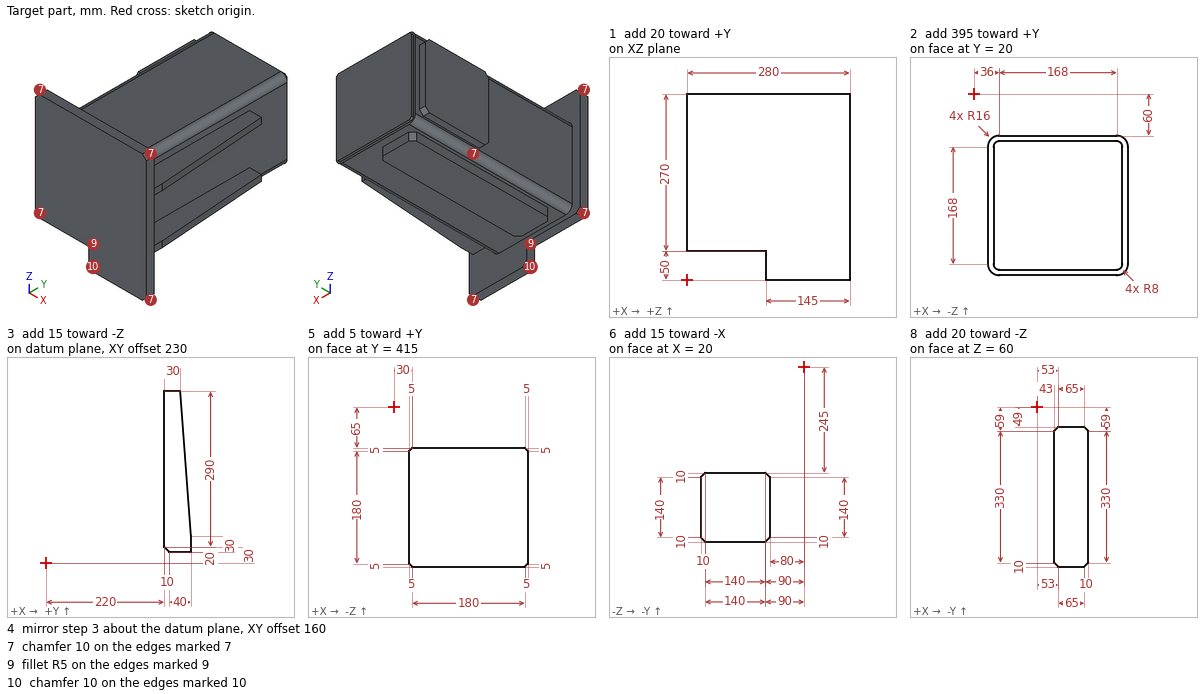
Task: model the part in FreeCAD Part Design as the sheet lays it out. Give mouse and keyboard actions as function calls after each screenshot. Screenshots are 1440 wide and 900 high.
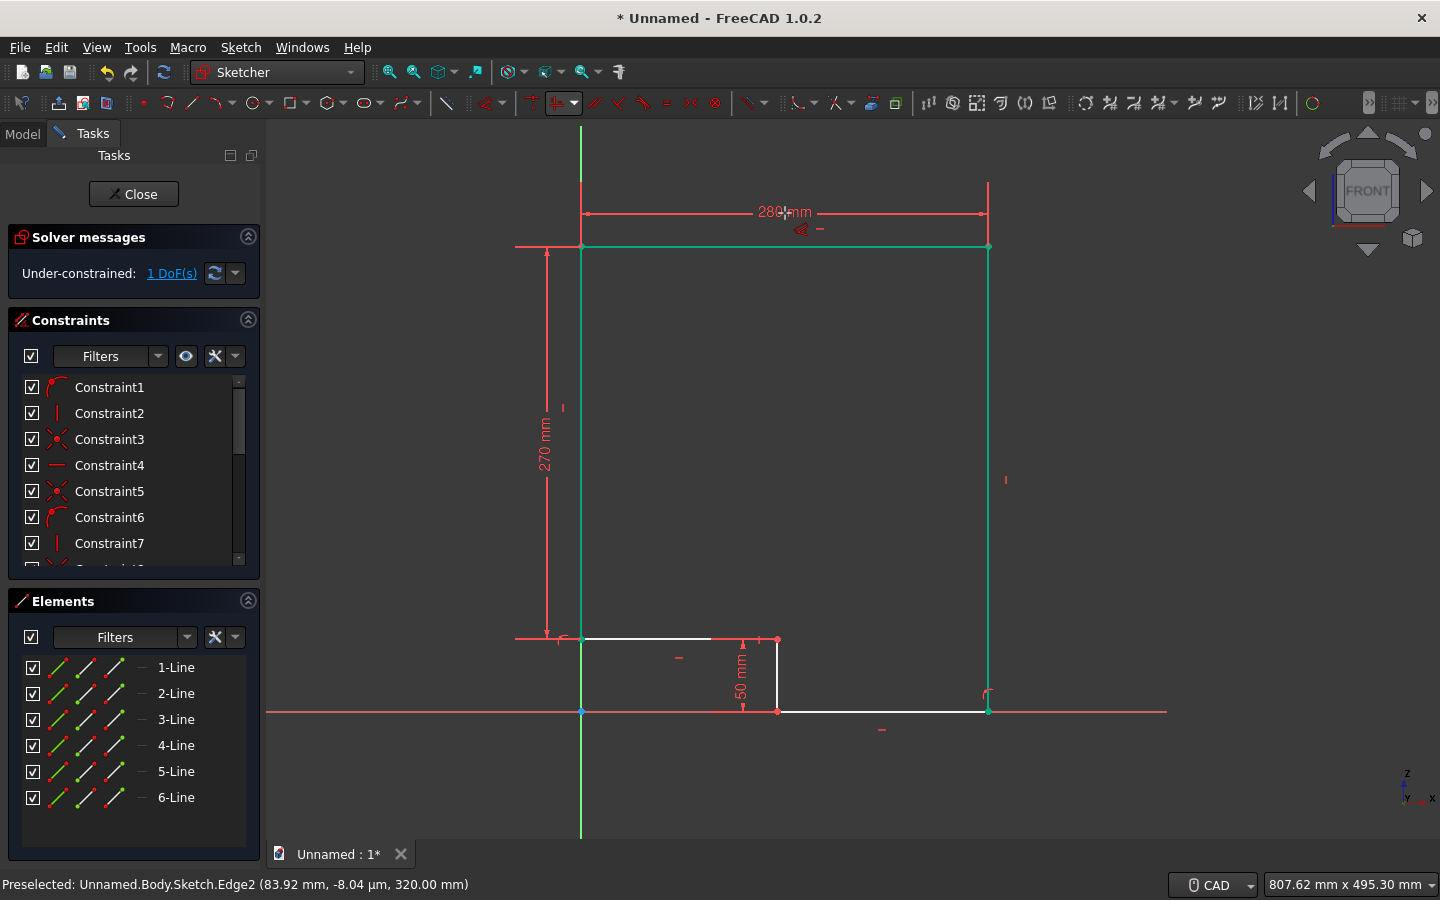
click(925, 712)
click(883, 746)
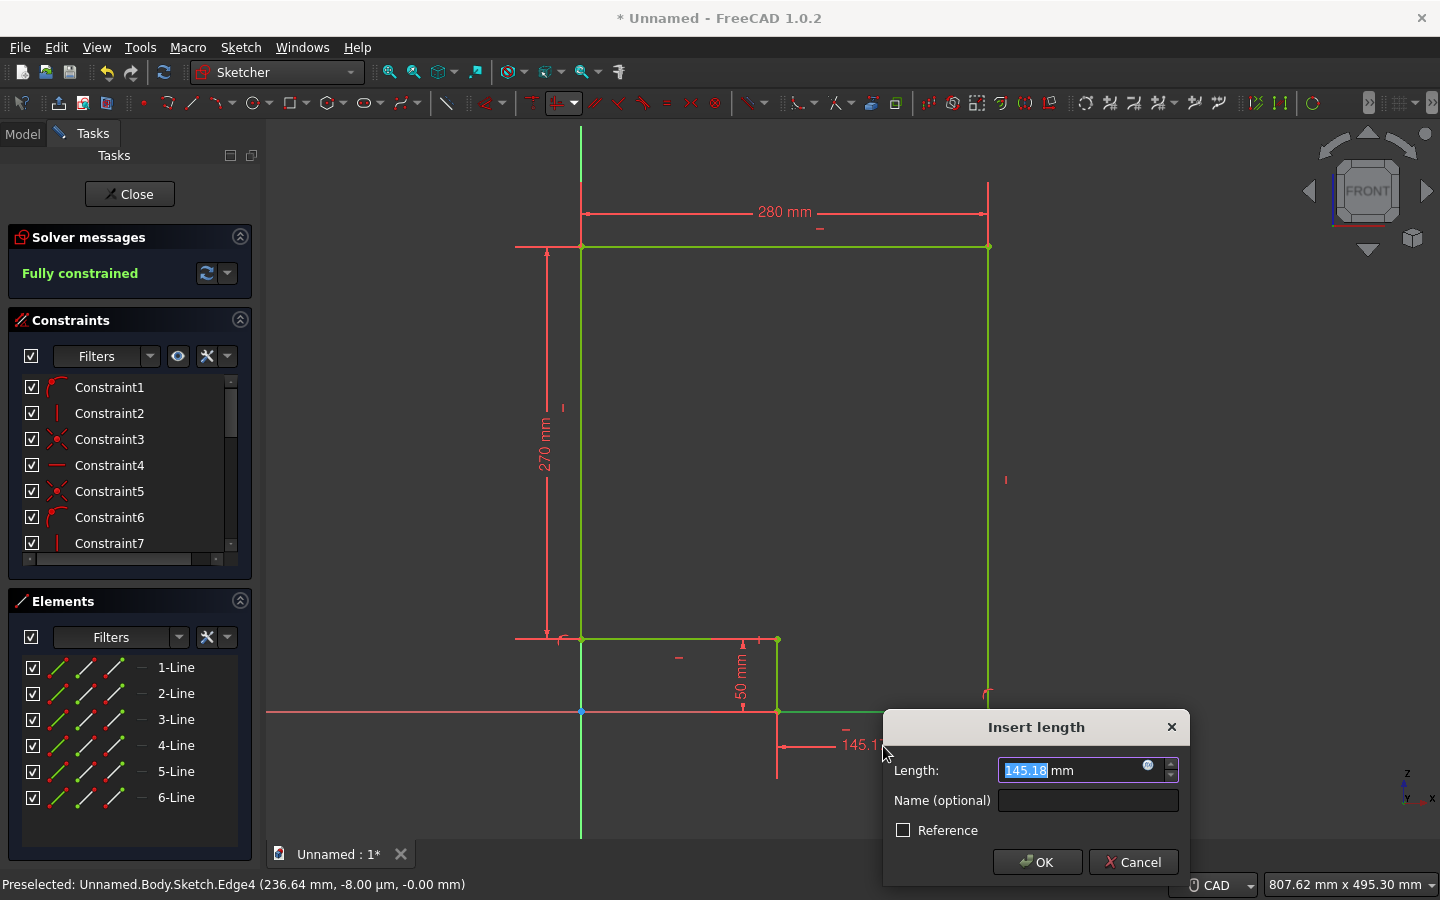
text(145)
key(Return)
key(Escape)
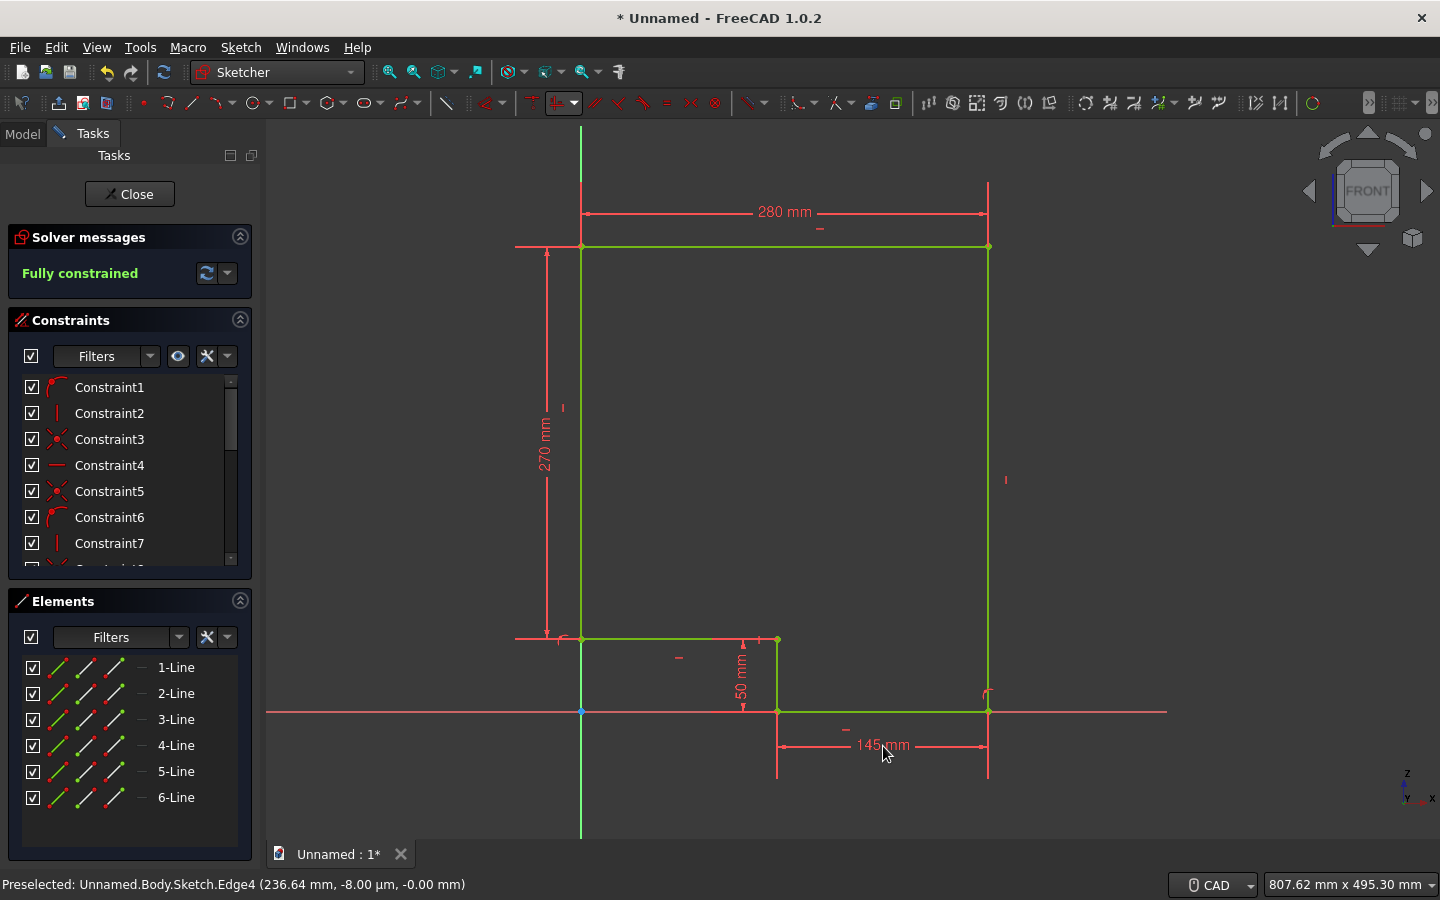
click(130, 194)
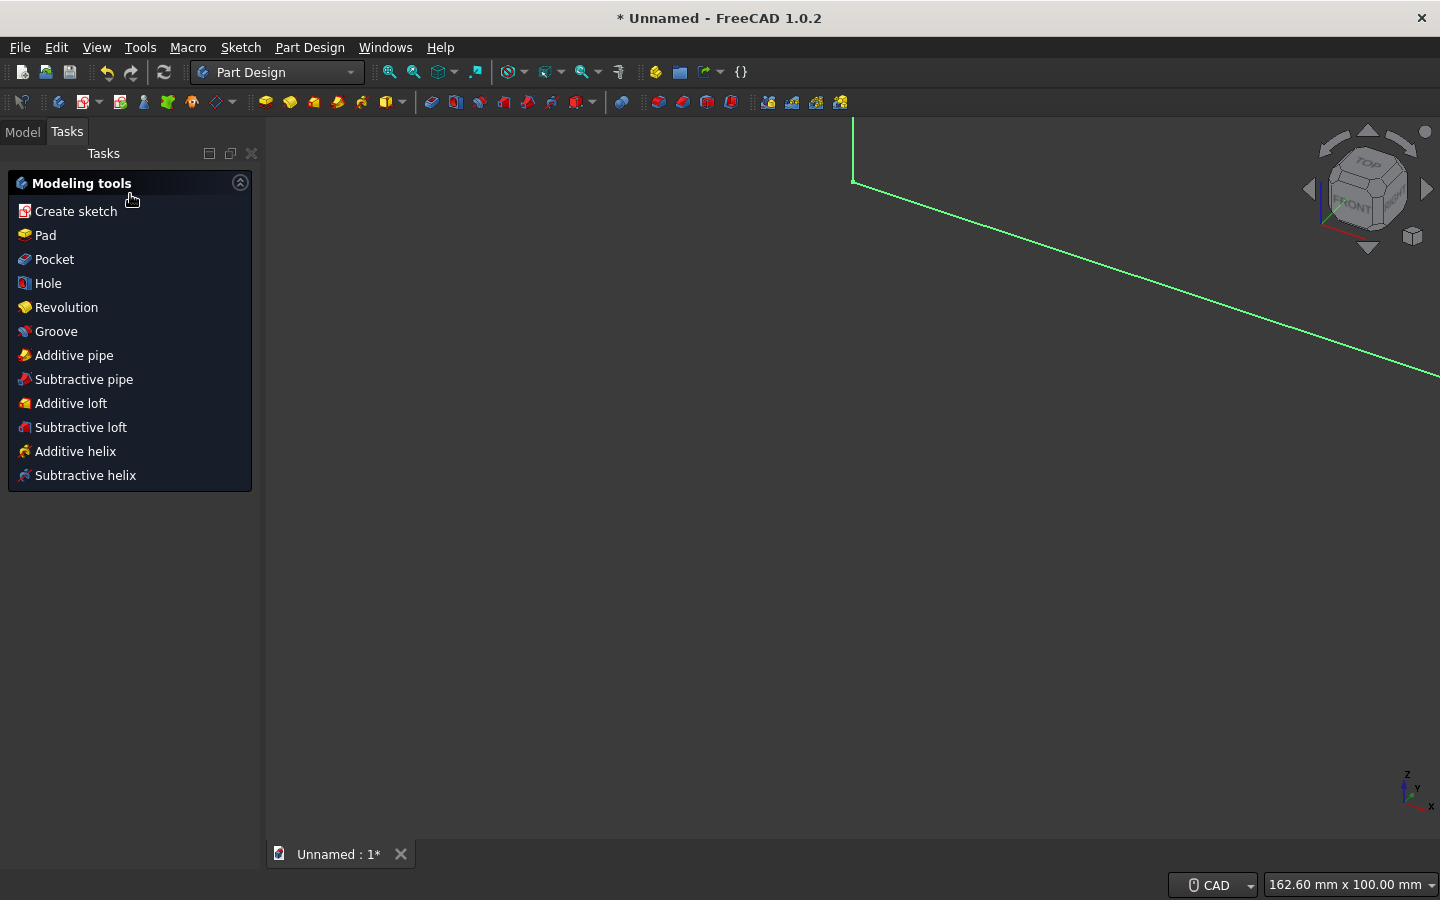
click(266, 102)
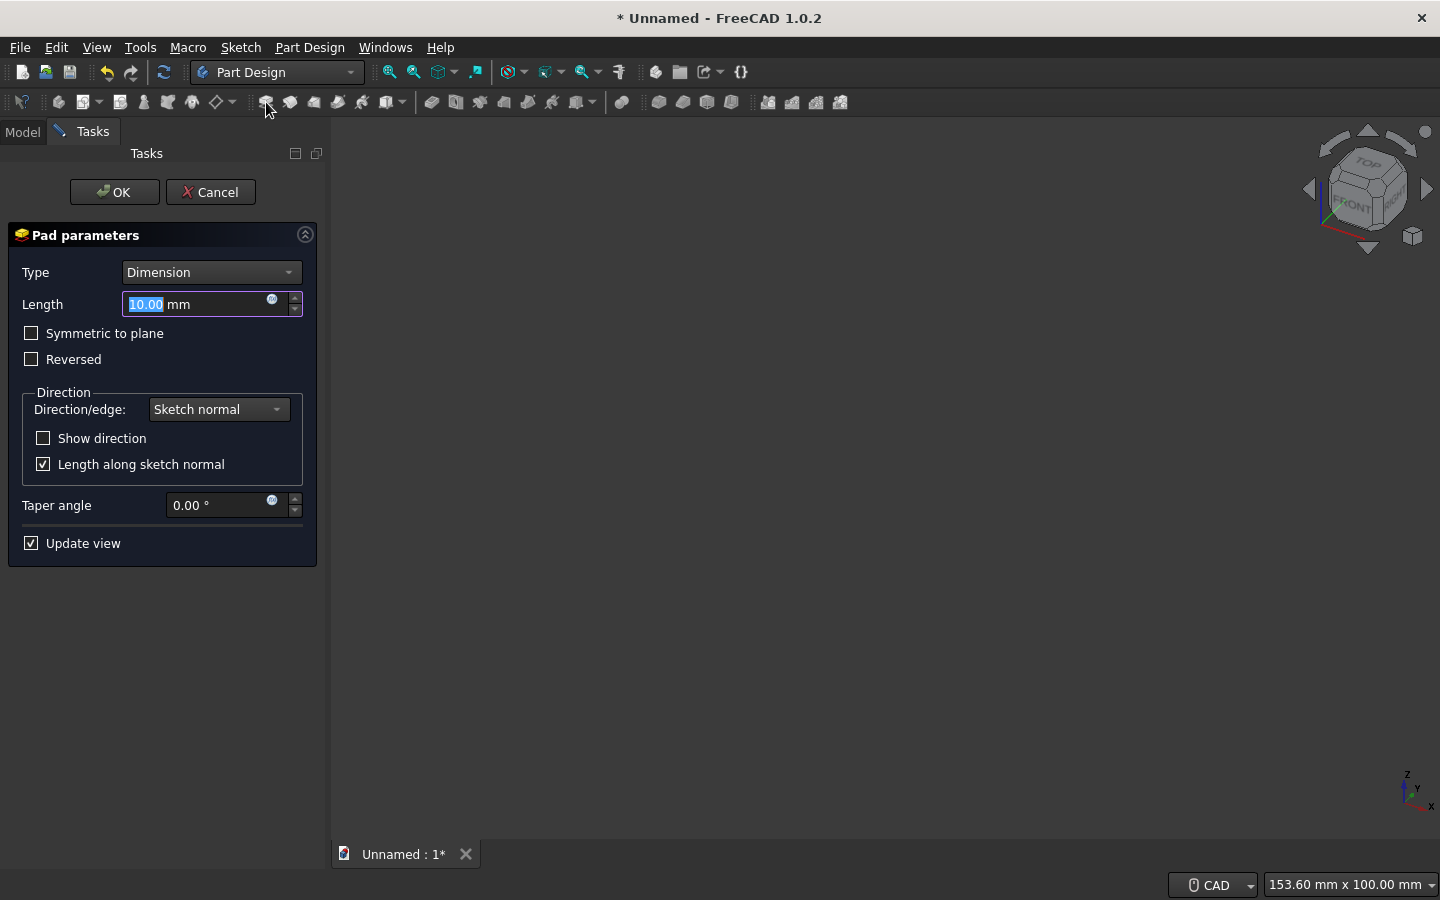
text(20)
key(Tab)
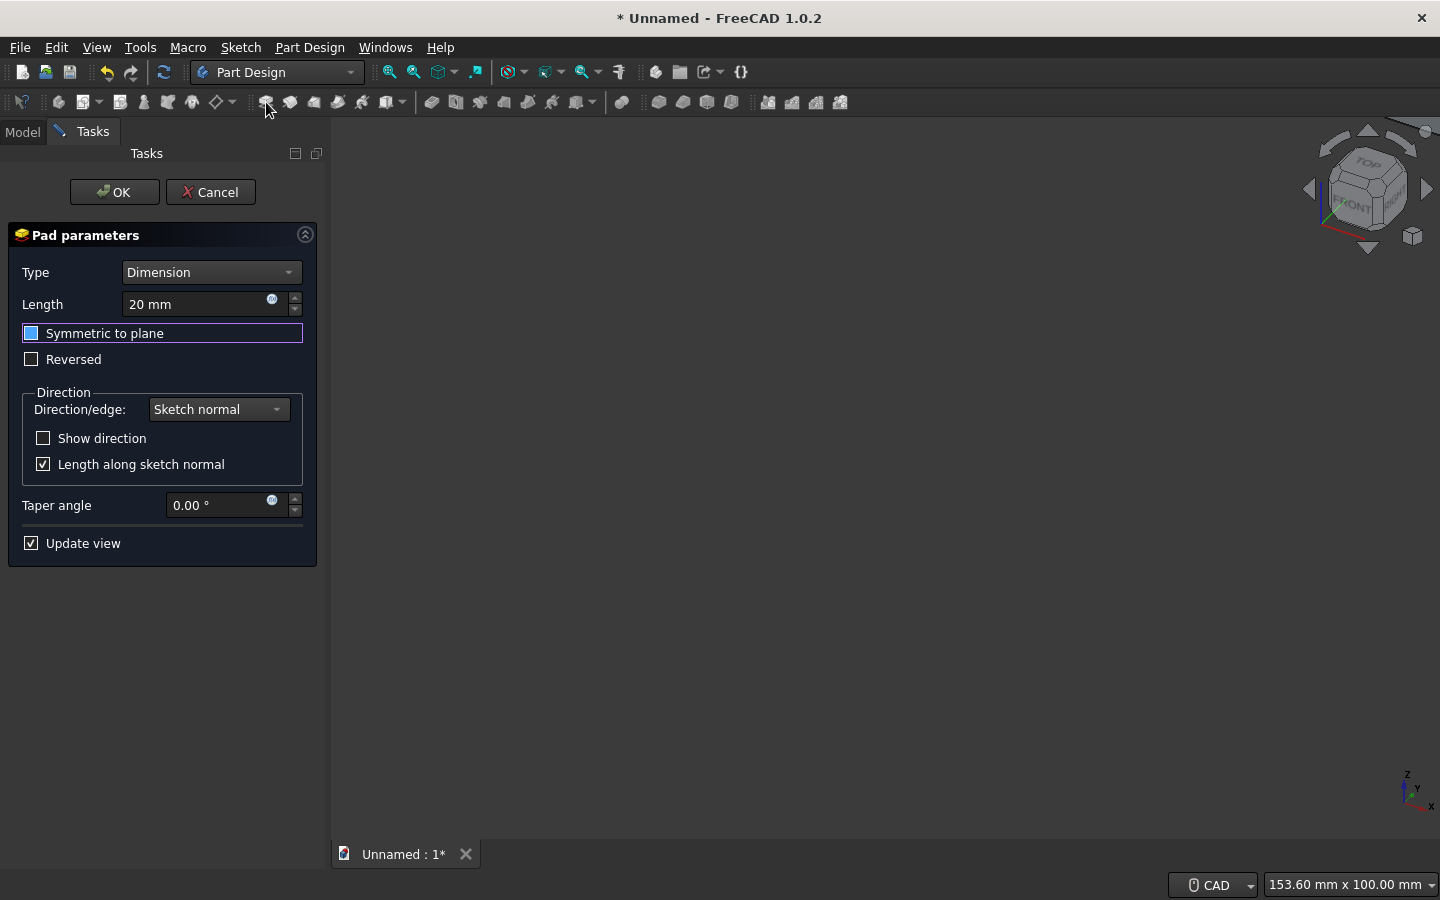
click(30, 359)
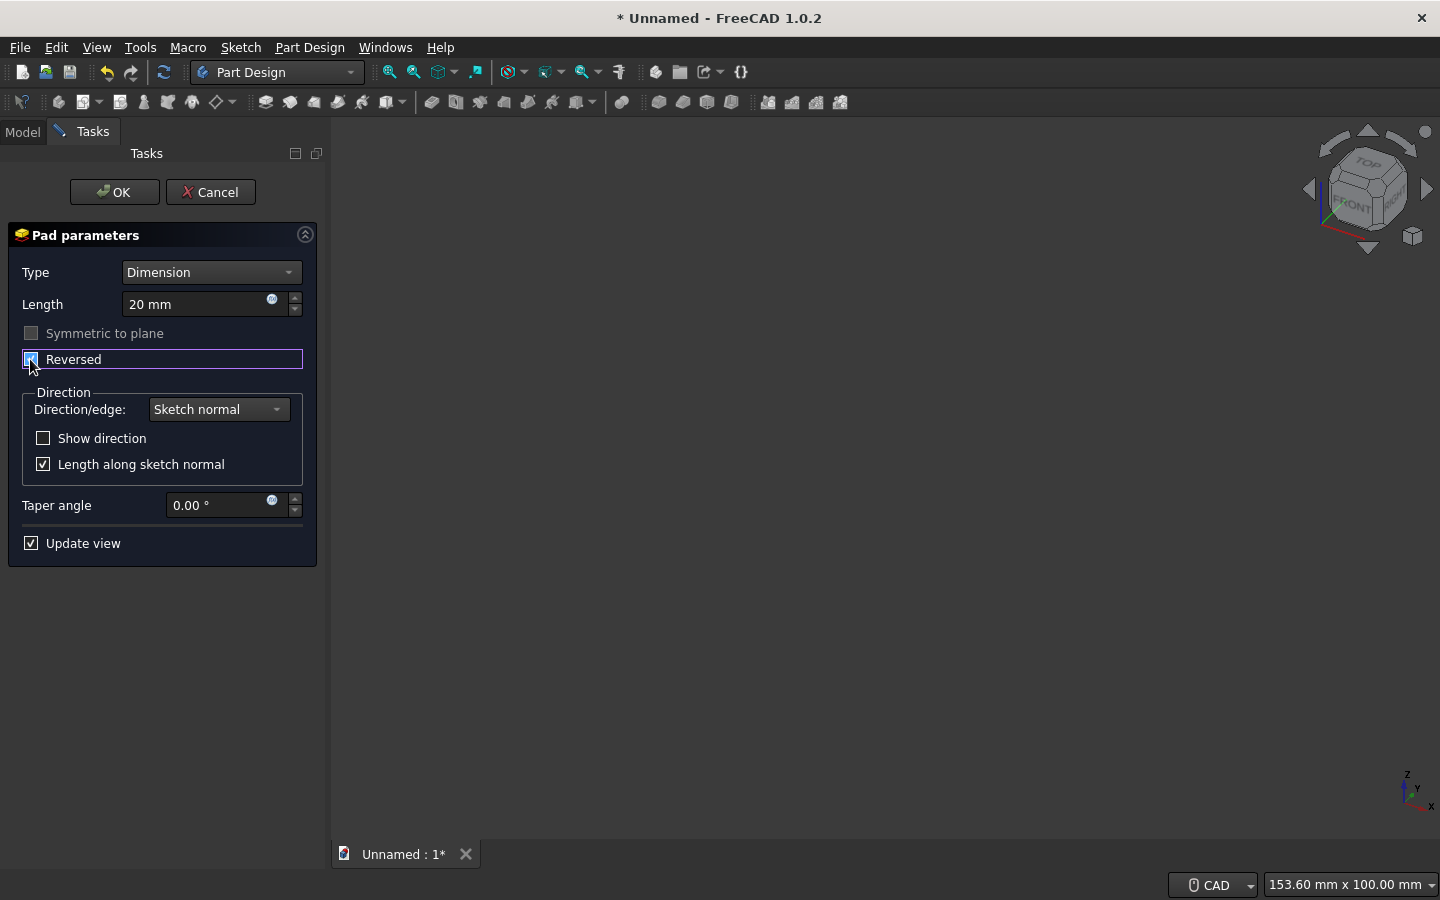
click(115, 192)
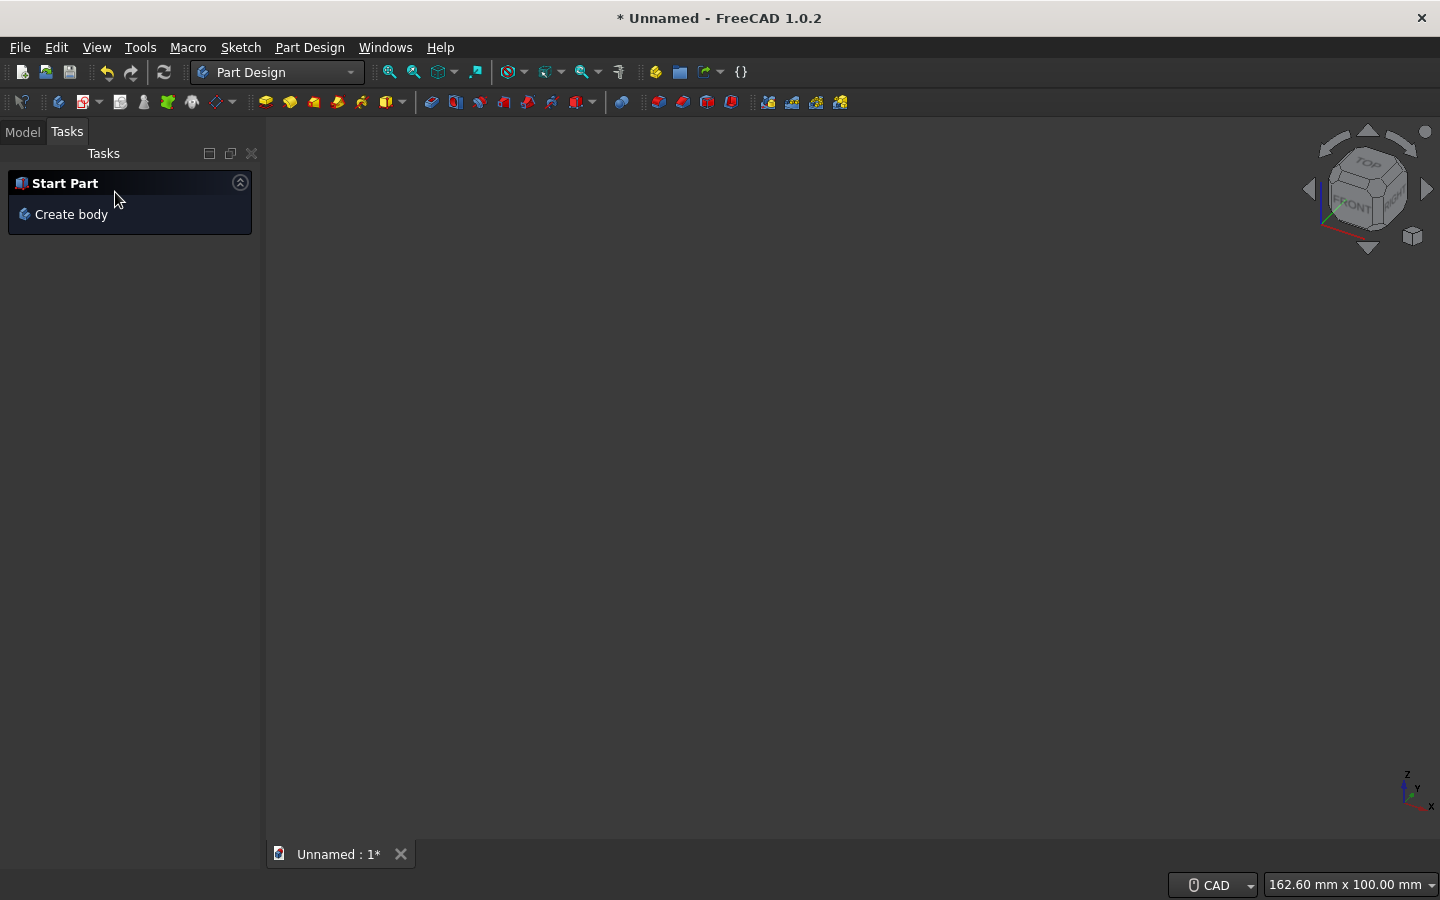
click(390, 72)